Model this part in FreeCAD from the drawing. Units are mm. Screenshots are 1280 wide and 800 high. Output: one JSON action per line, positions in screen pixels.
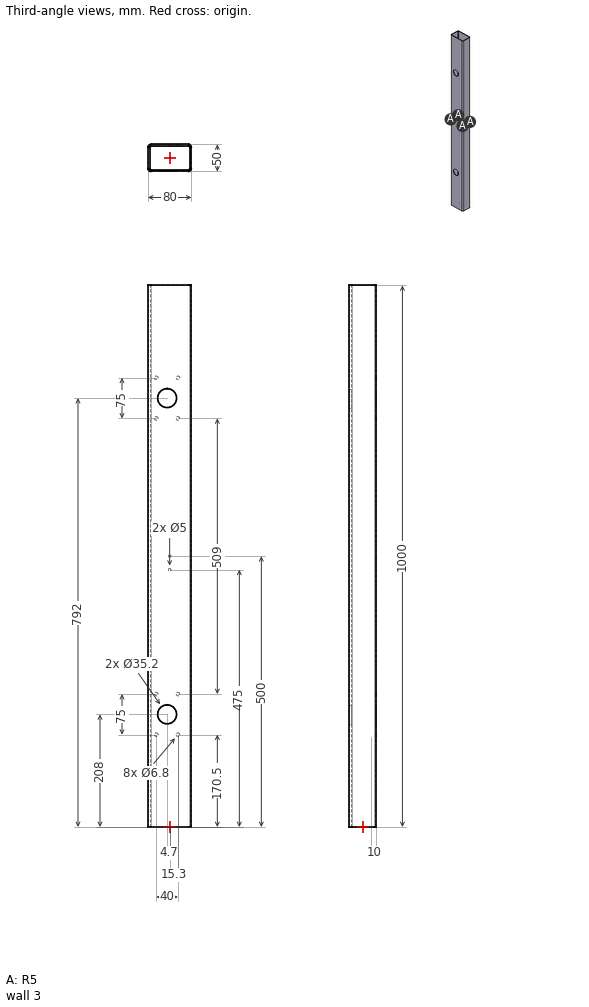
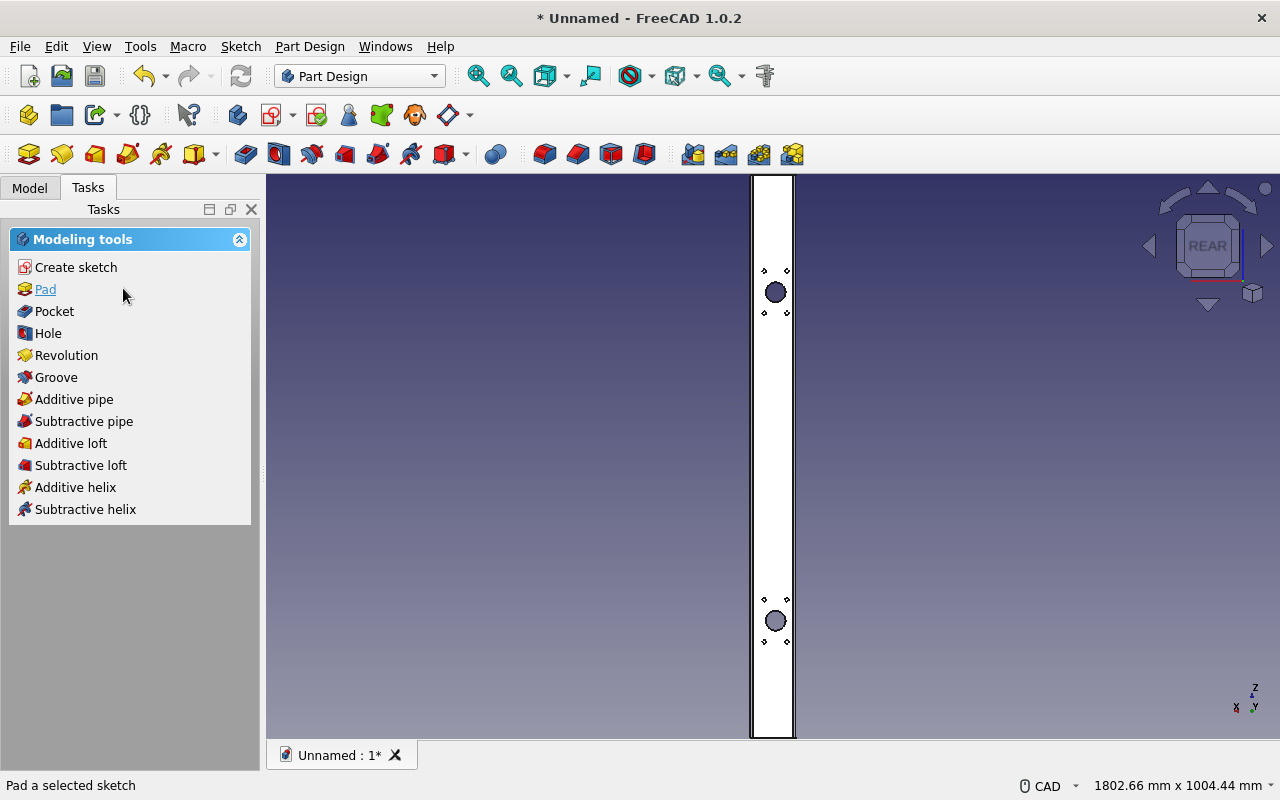
{"action": "left_click", "coordinate": [246, 154]}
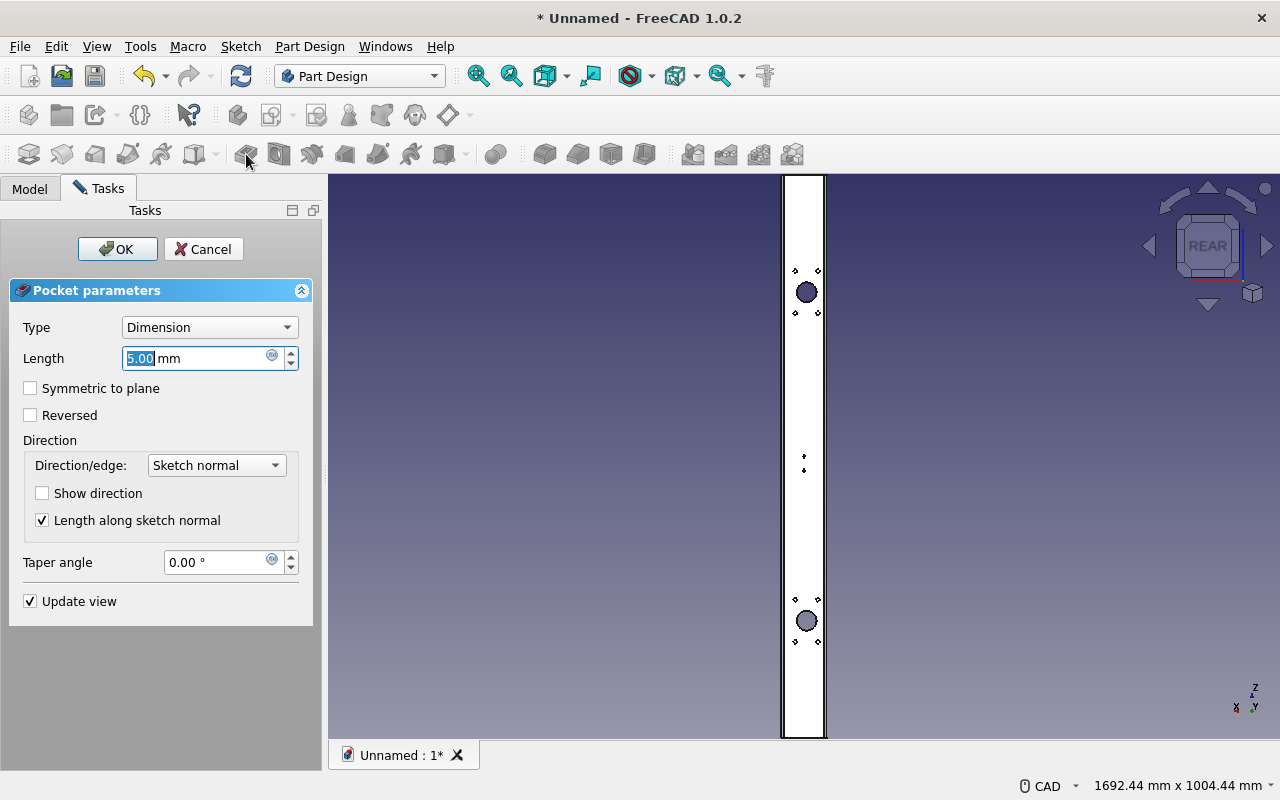
{"action": "type", "text": "10"}
{"action": "key", "text": "Tab"}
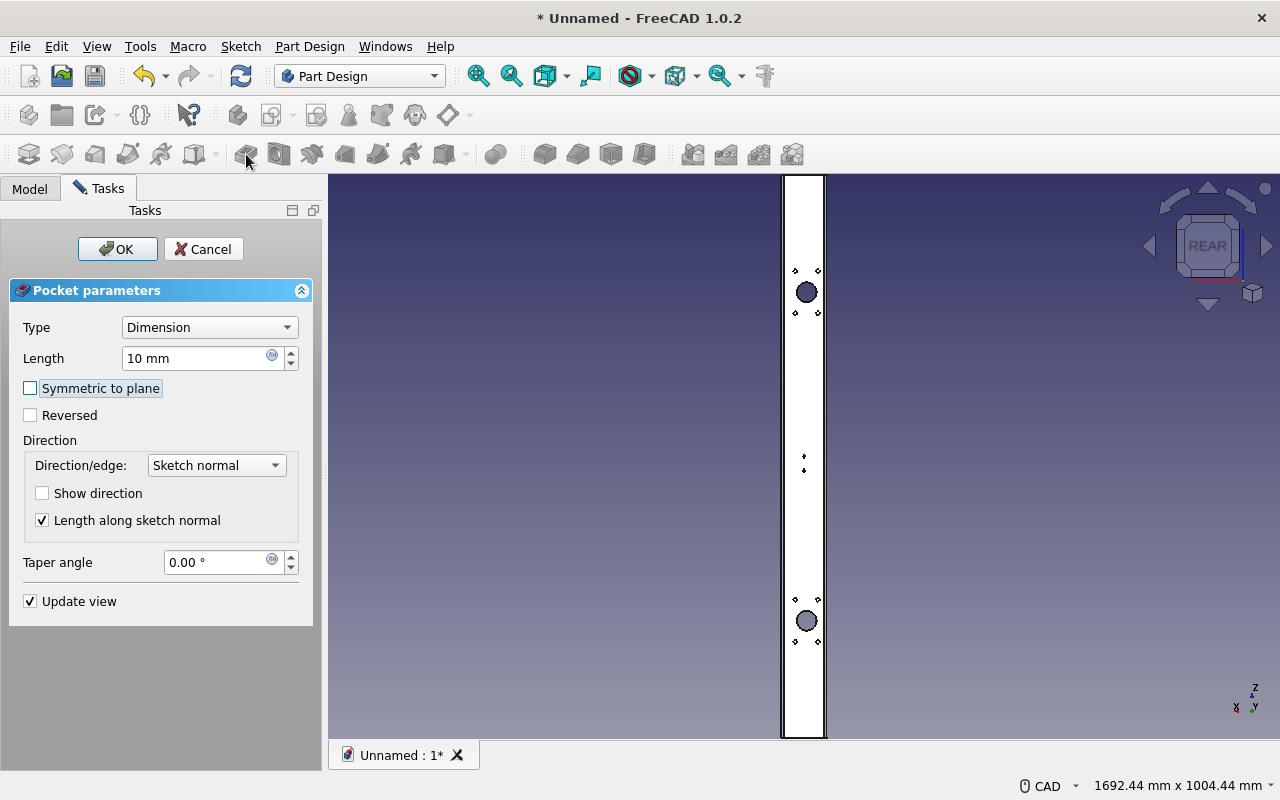
{"action": "left_click", "coordinate": [118, 249]}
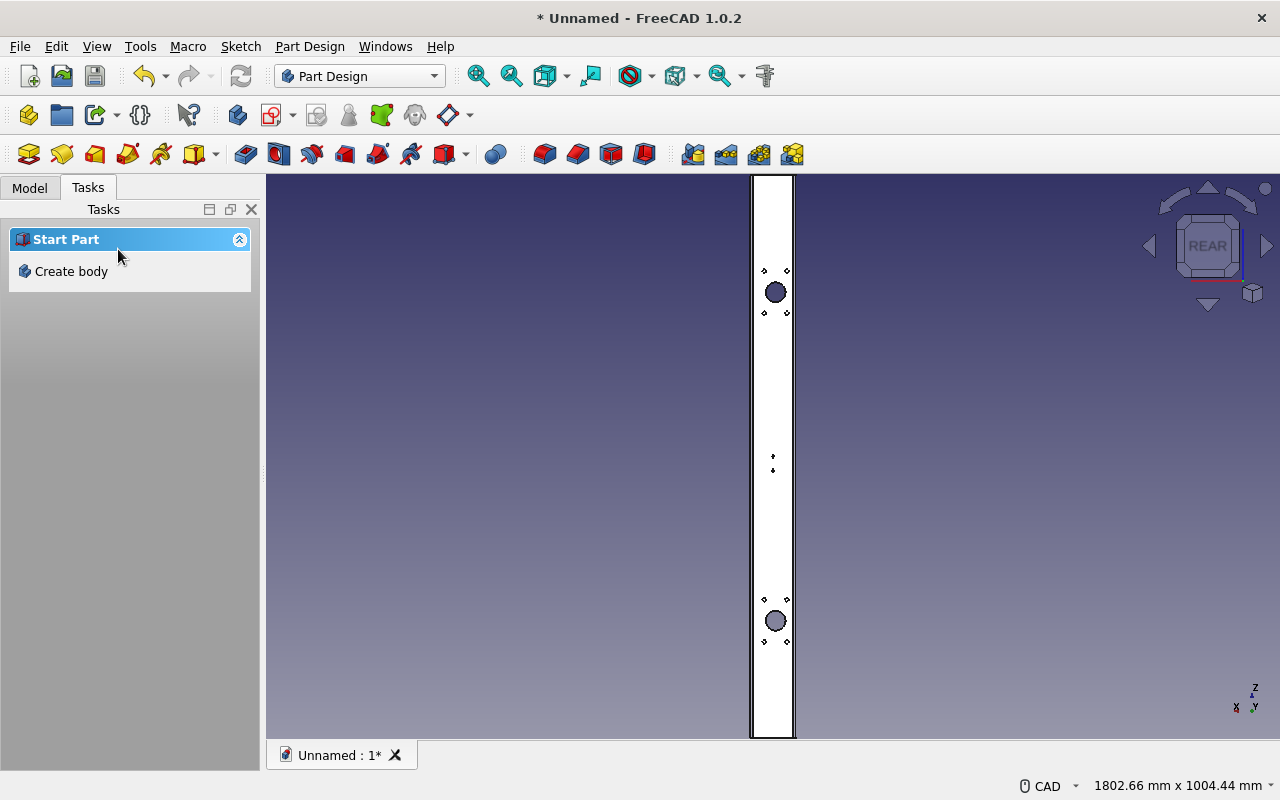
{"action": "key", "text": "0"}